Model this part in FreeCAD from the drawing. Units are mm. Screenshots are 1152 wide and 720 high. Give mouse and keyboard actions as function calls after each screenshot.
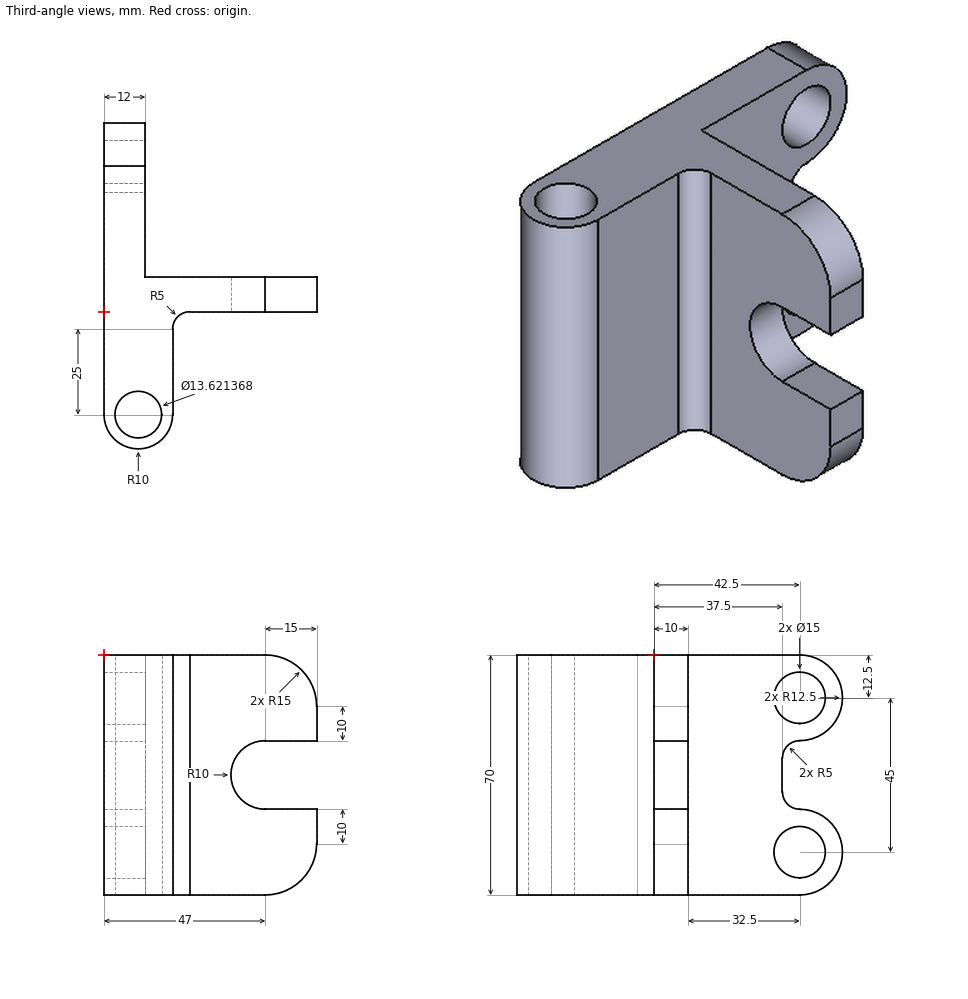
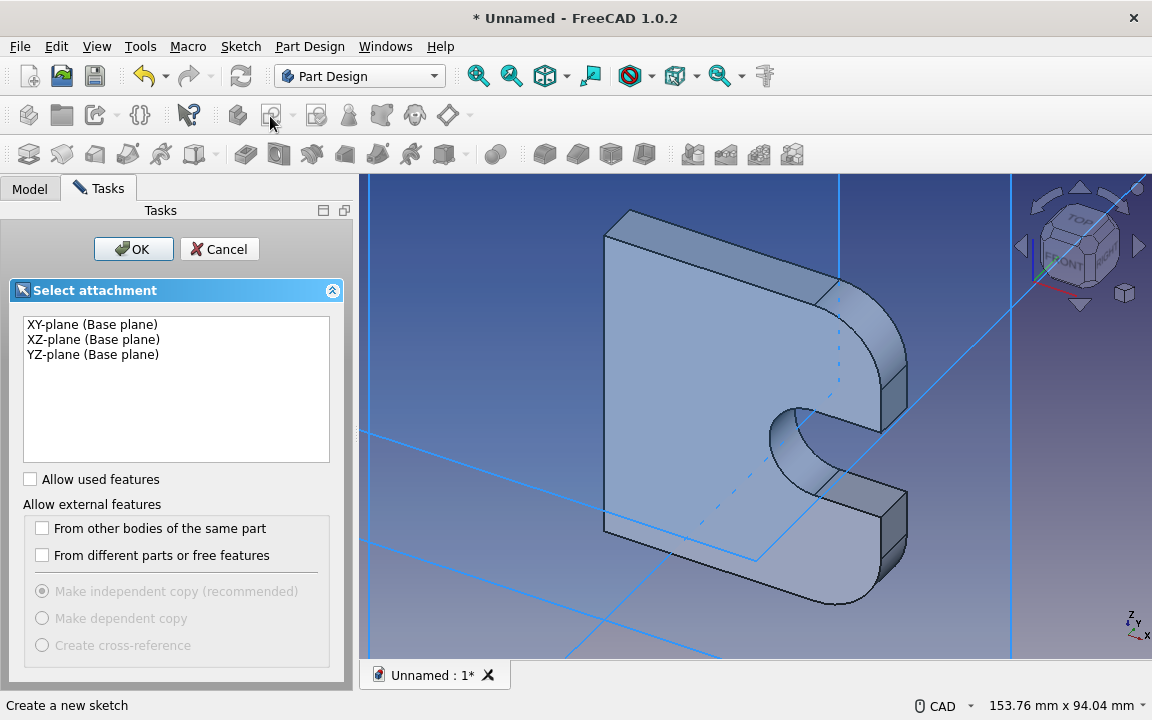
click(84, 324)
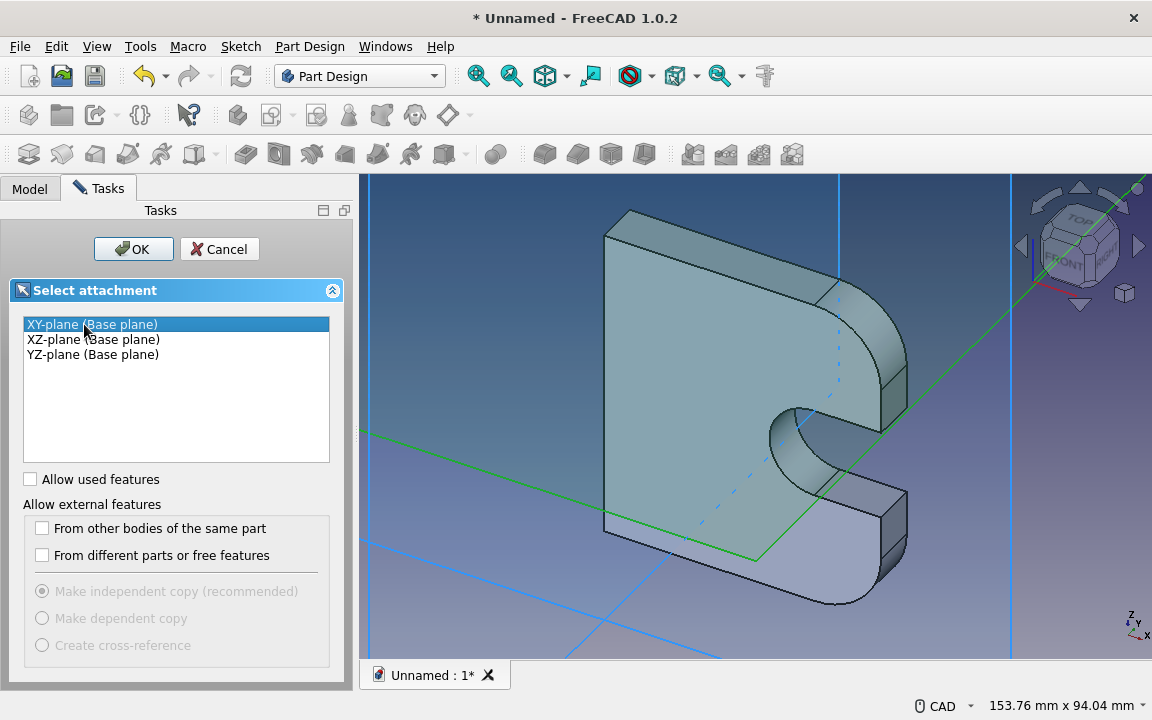
click(134, 249)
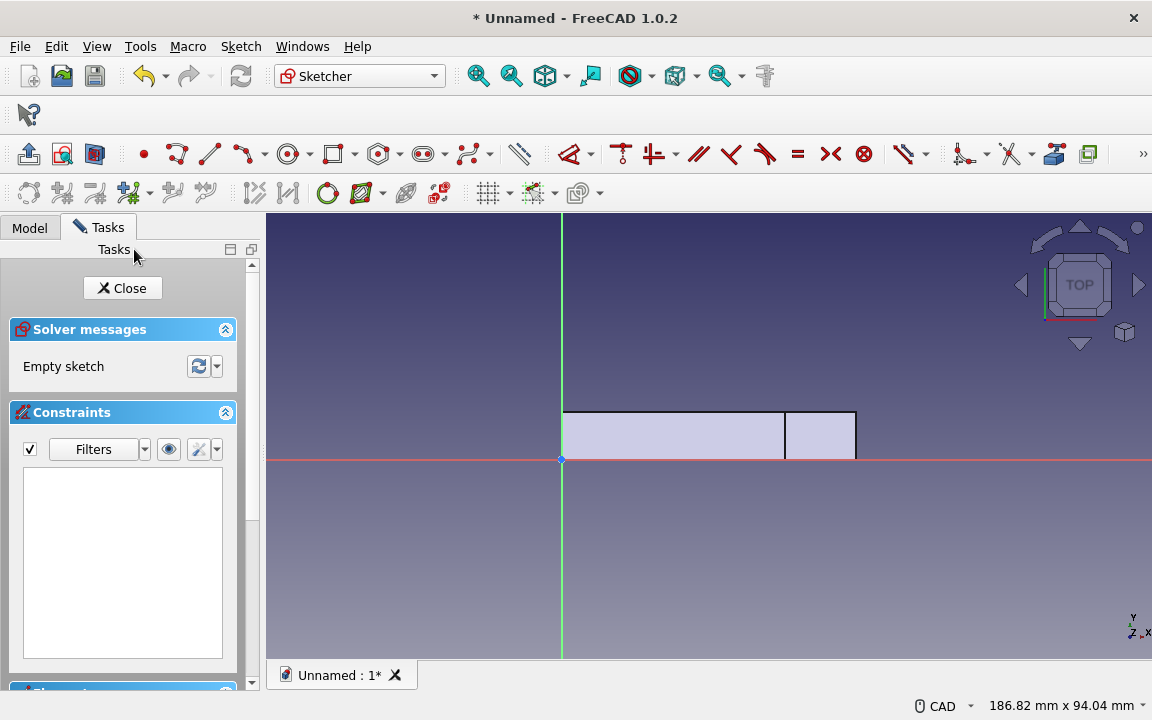
scroll(727, 241, down, 1)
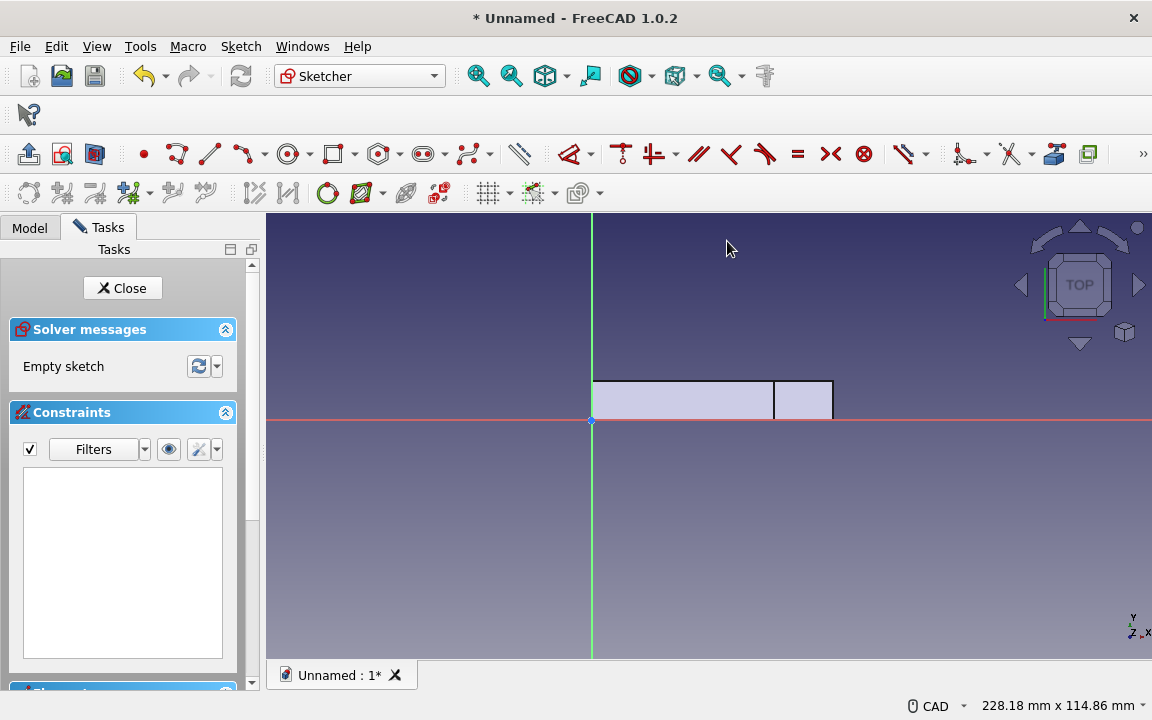
scroll(641, 573, up, 3)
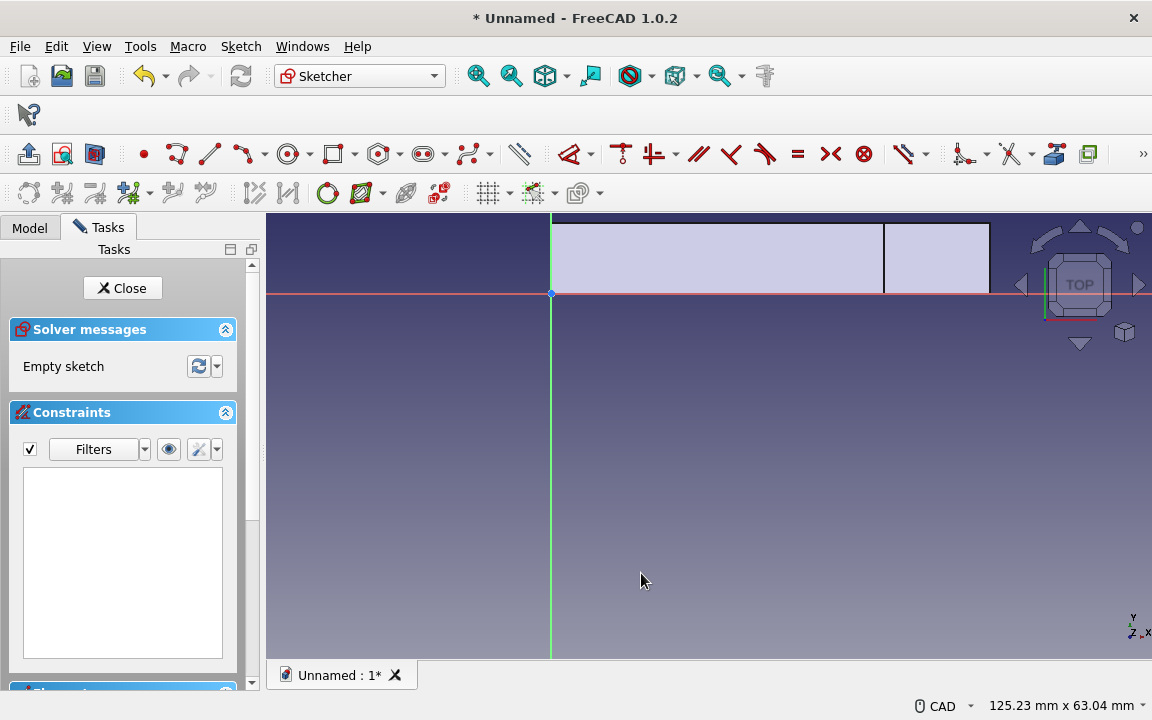
click(210, 154)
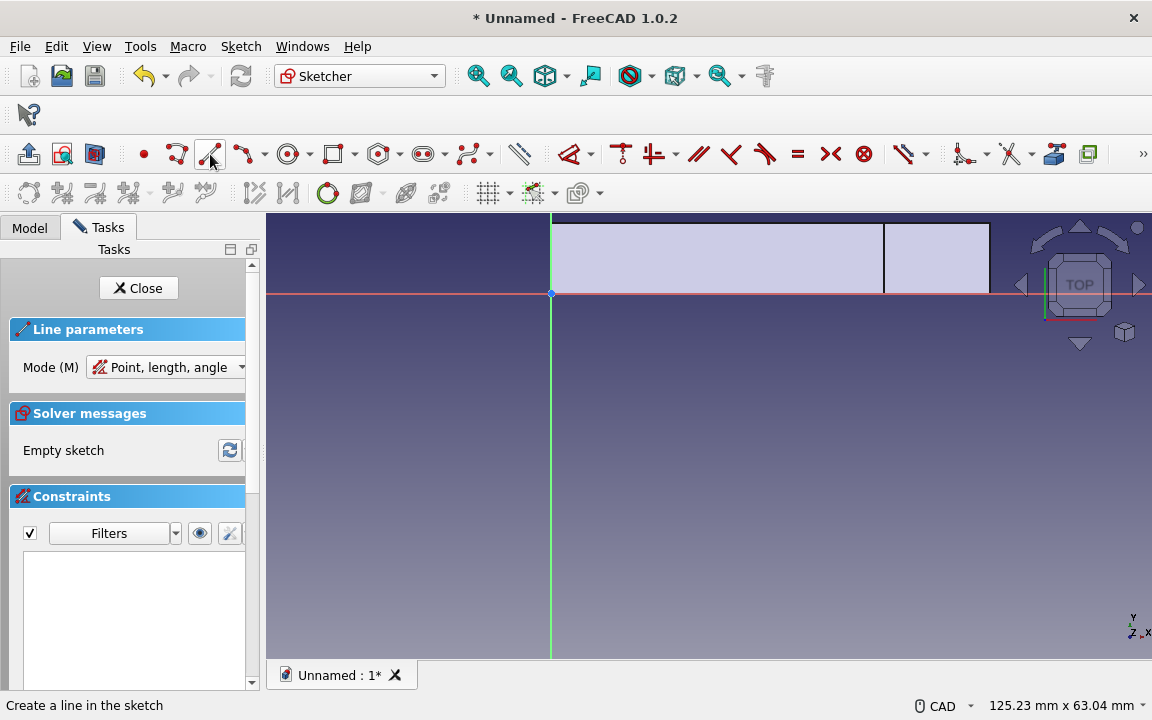
click(693, 506)
click(693, 329)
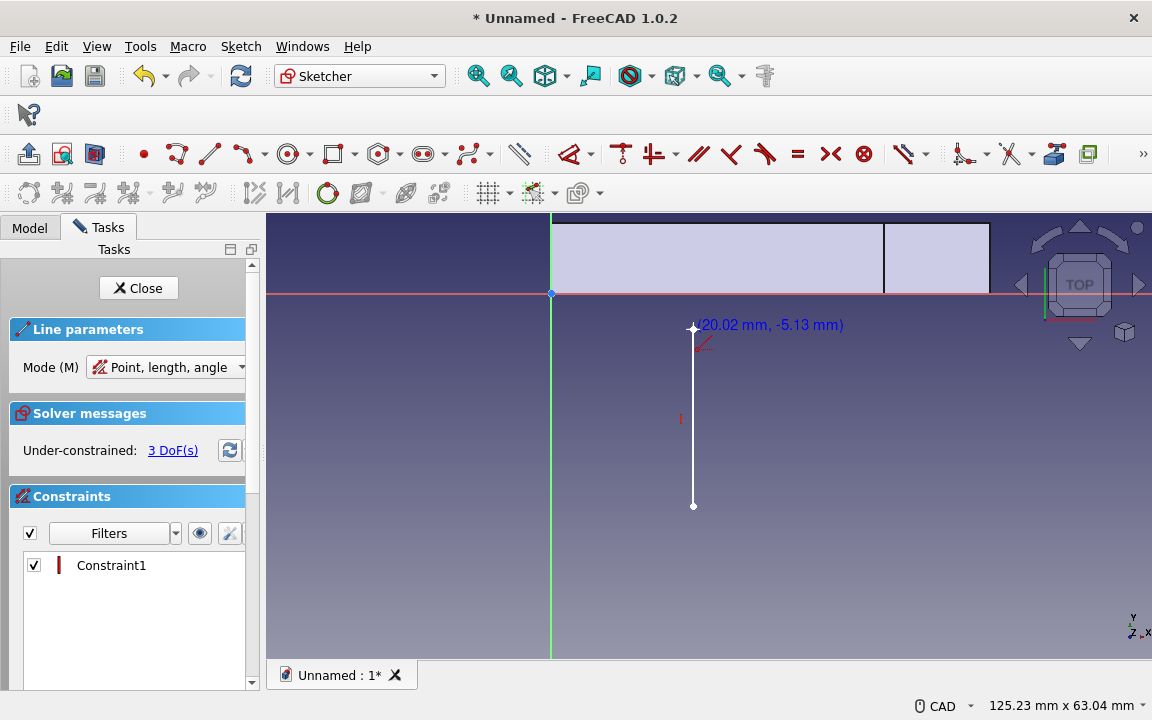
click(177, 154)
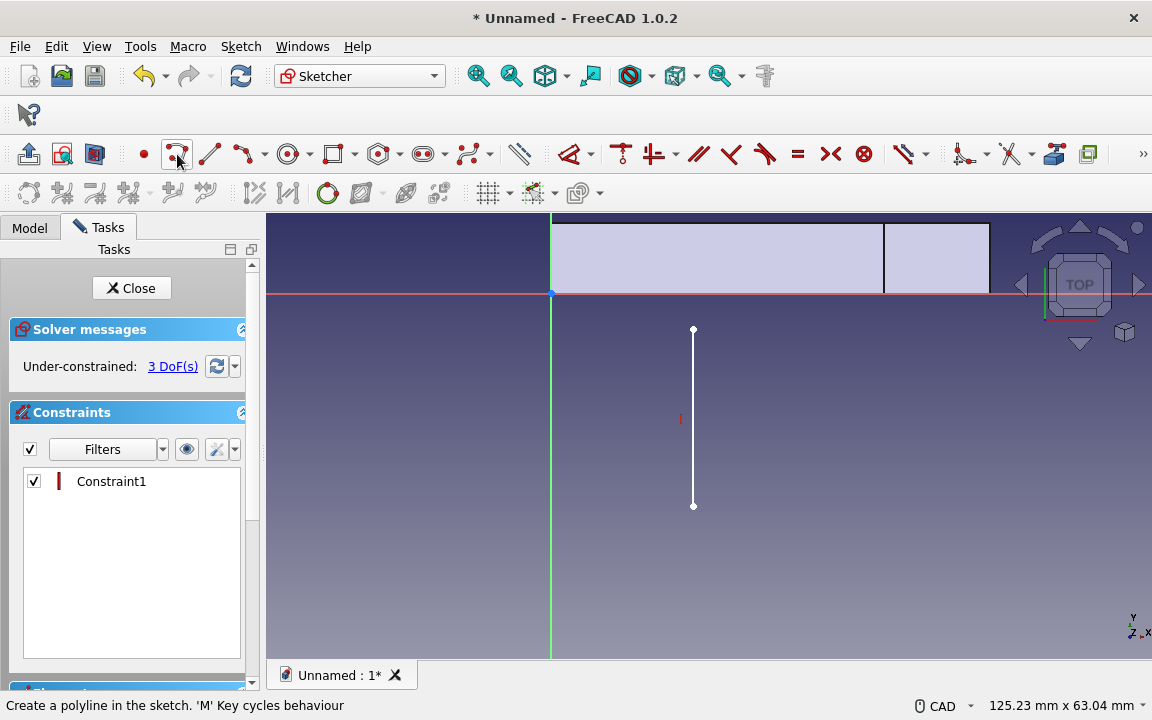
click(728, 294)
click(551, 294)
click(560, 506)
right_click(560, 506)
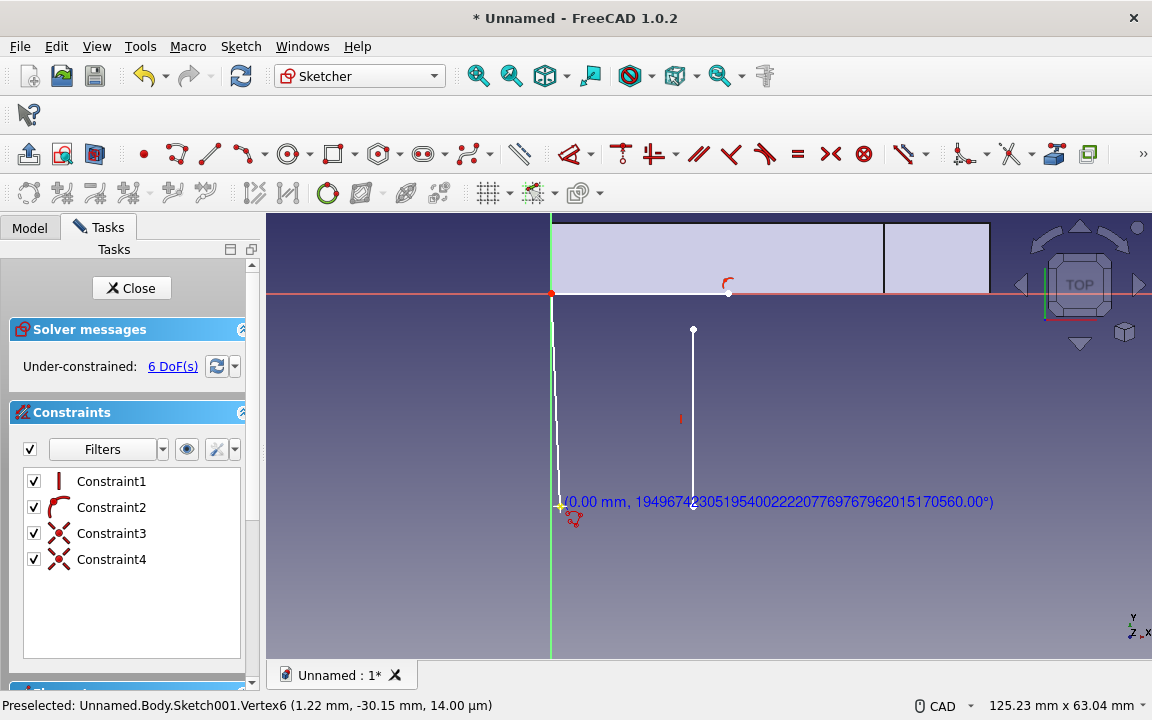
click(242, 154)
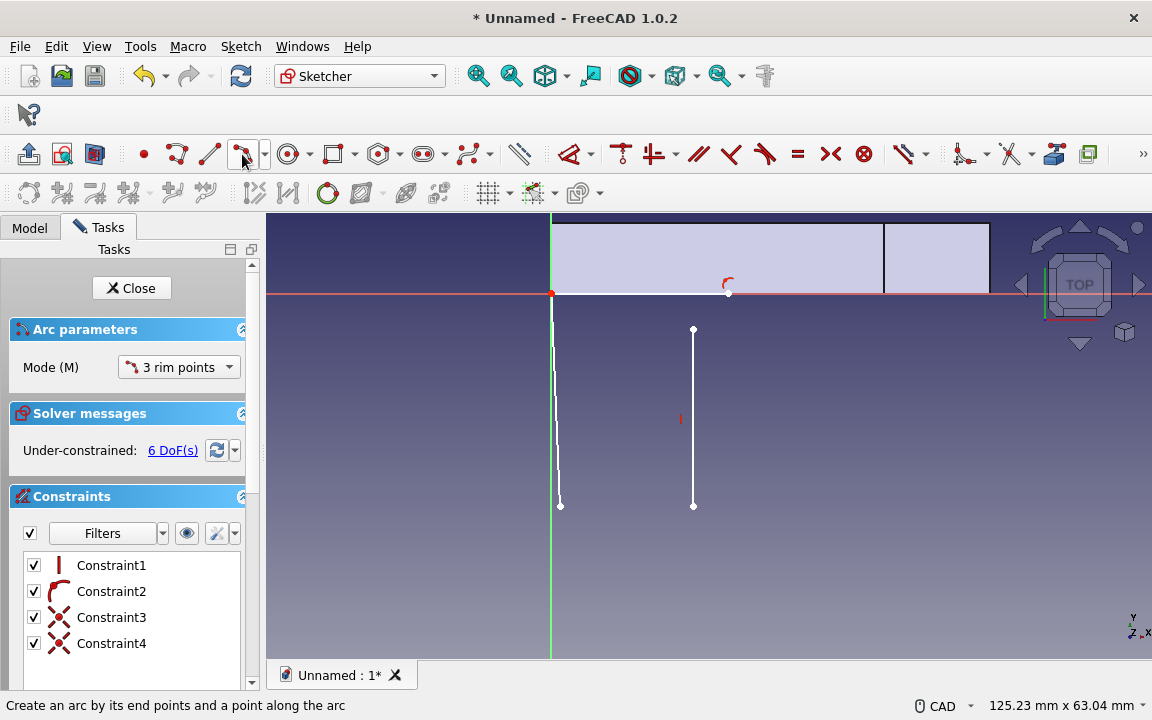
click(693, 330)
click(728, 294)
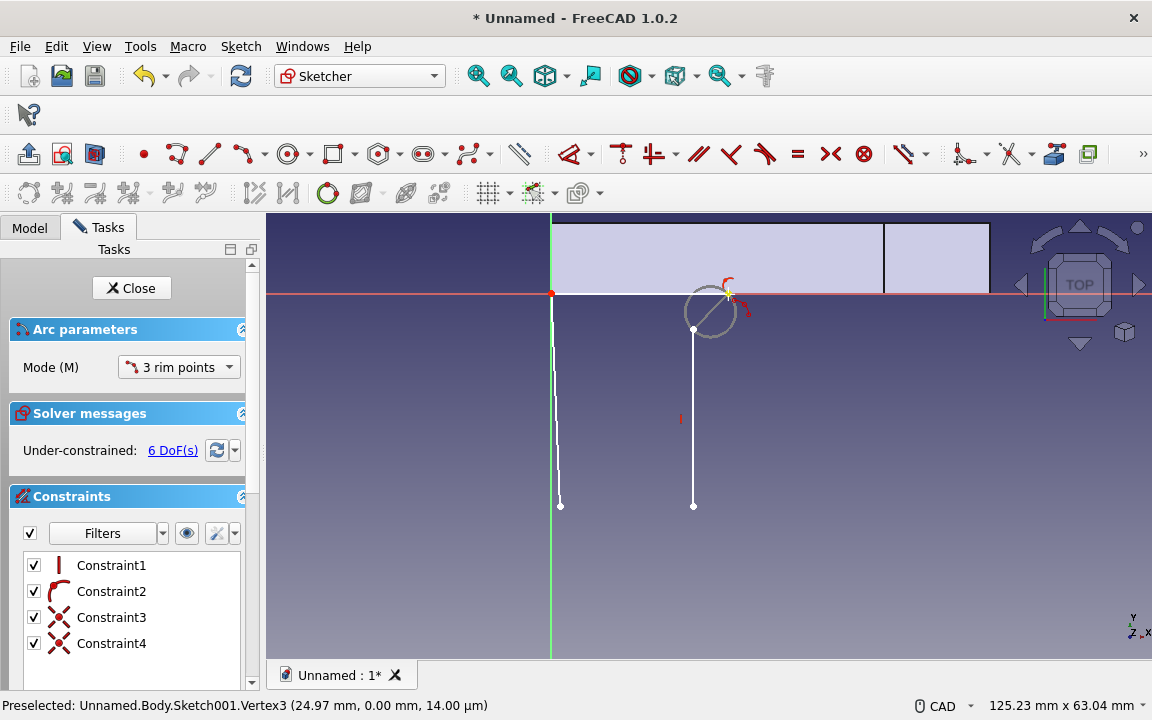
scroll(703, 304, up, 3)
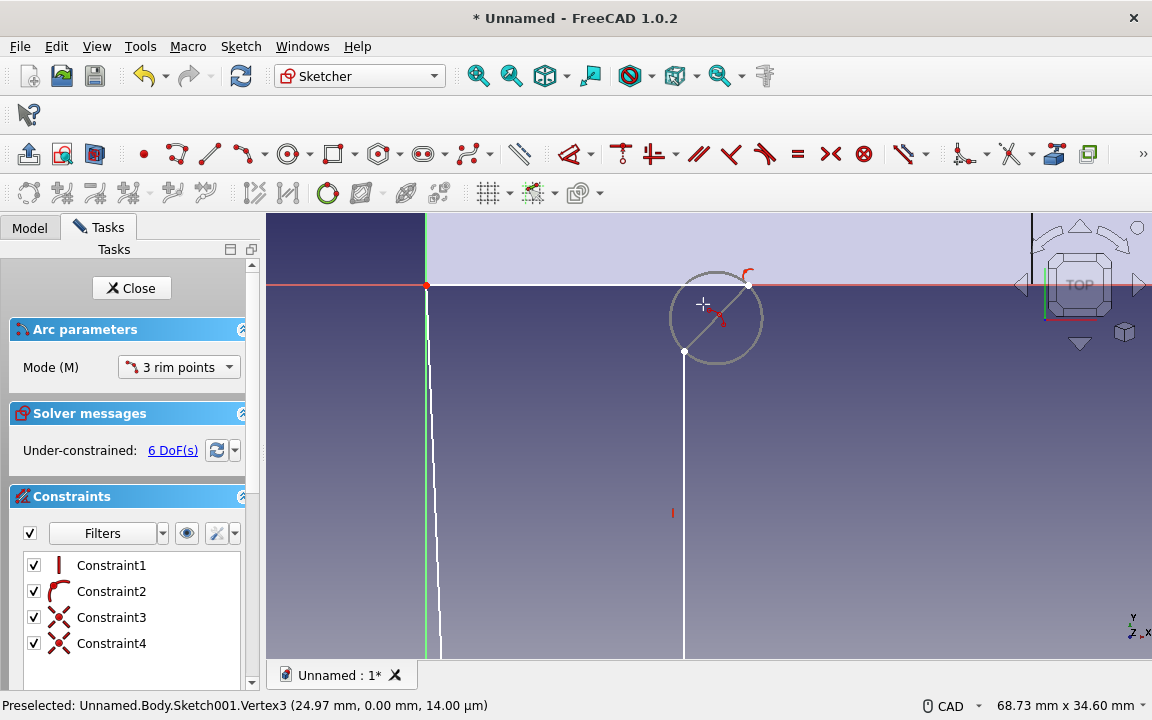
click(703, 304)